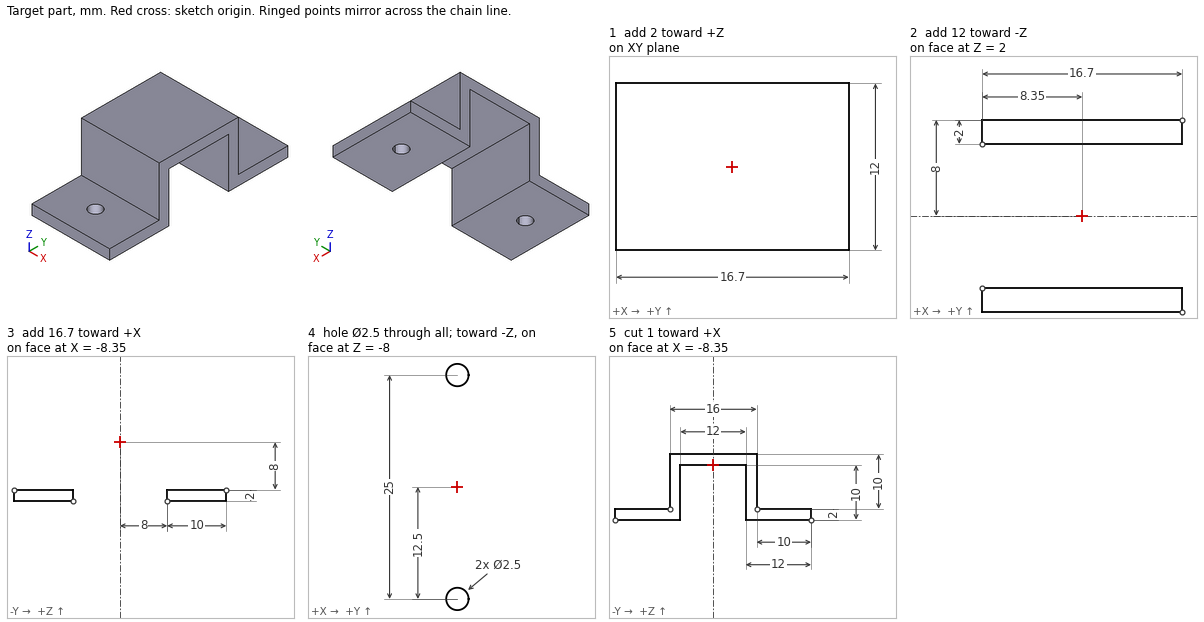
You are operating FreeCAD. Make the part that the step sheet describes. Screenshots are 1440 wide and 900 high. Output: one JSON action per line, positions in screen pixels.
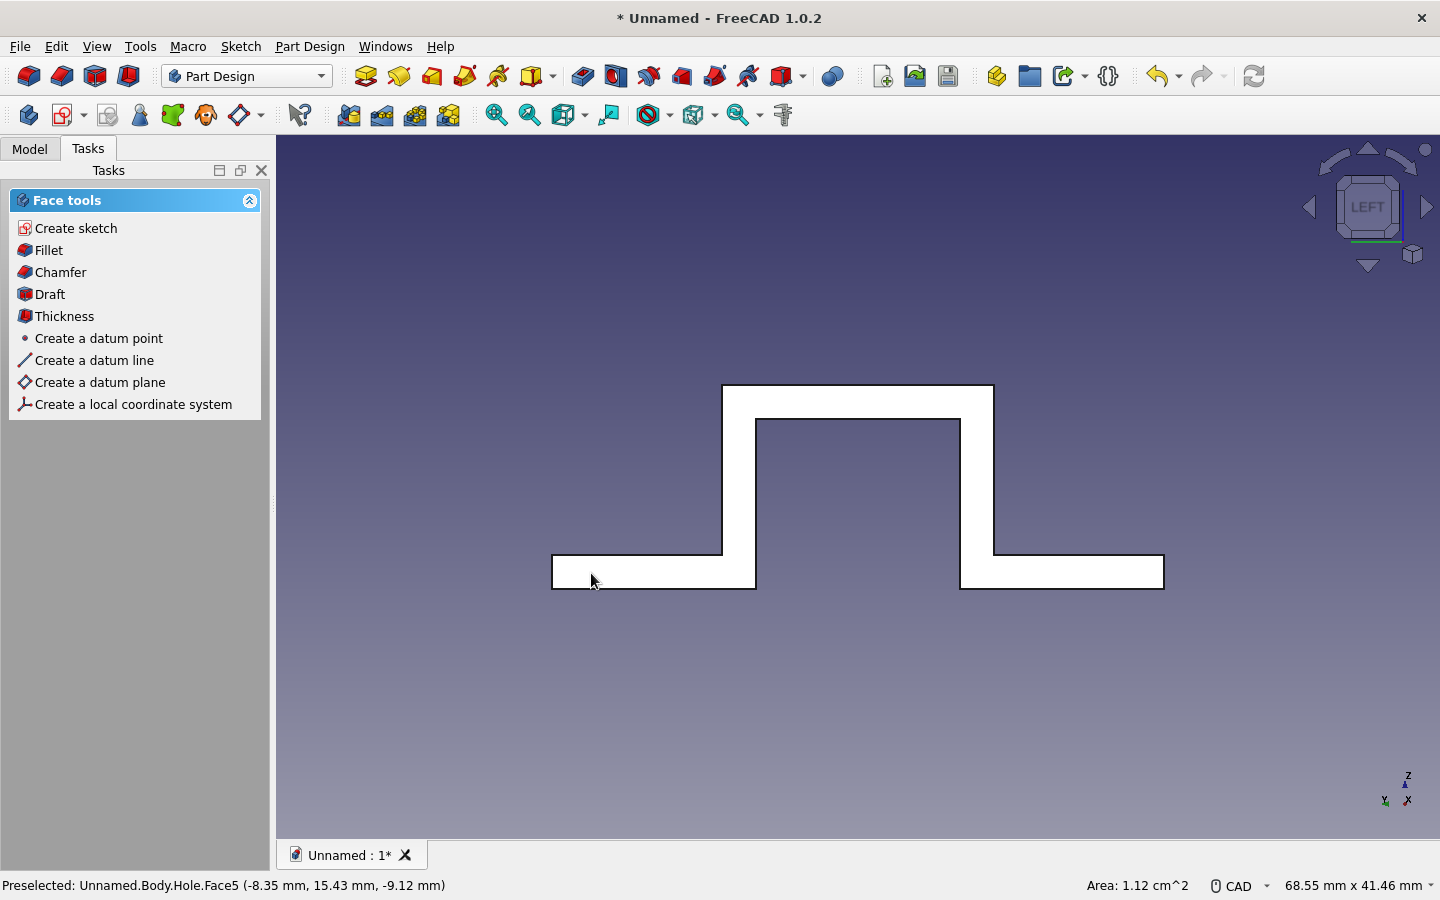
{"action": "left_click", "coordinate": [62, 116]}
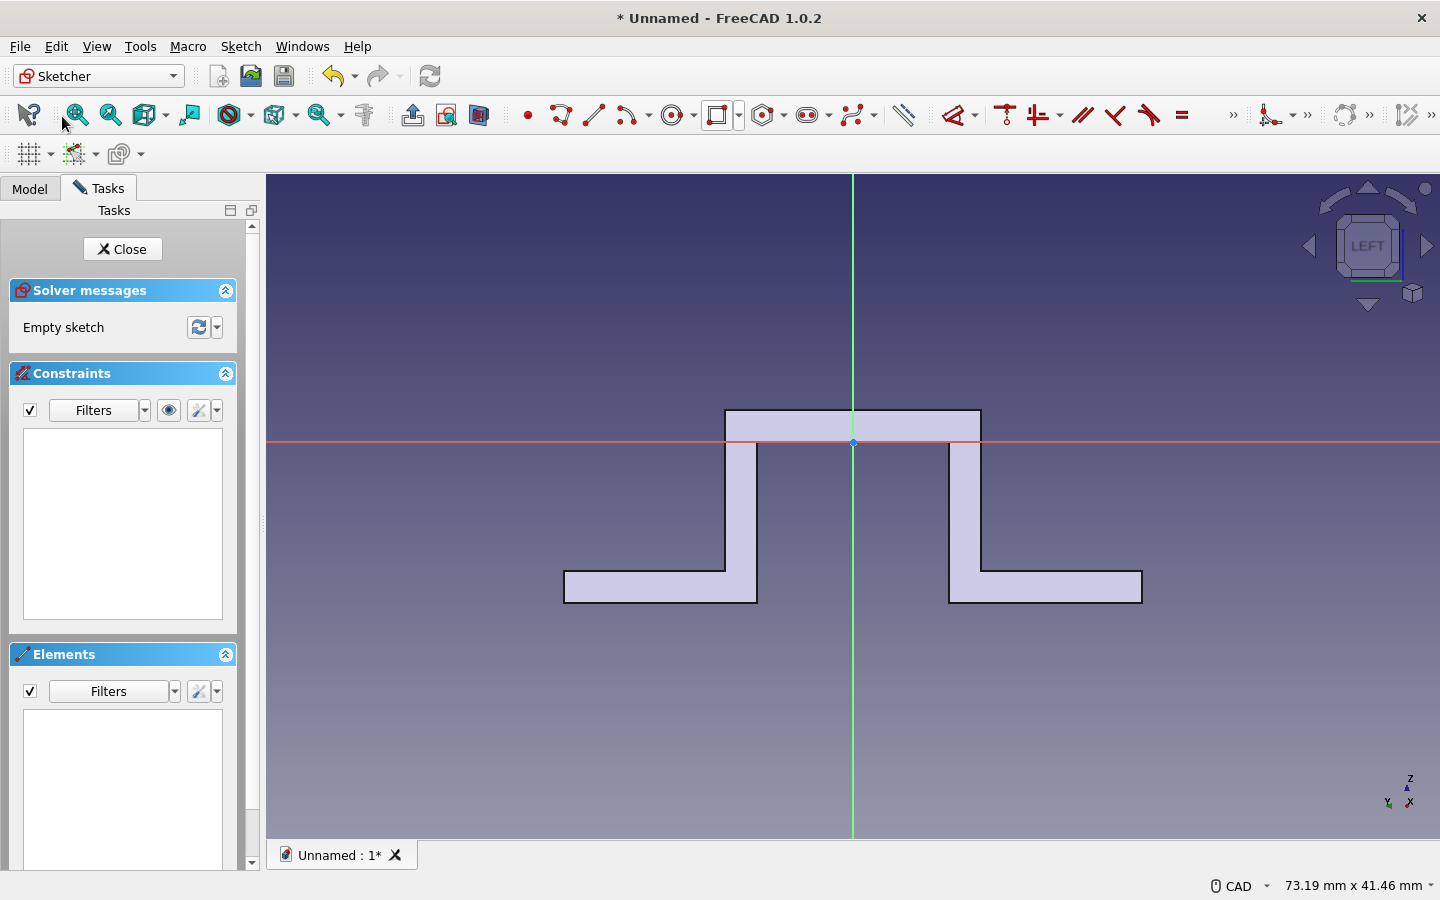
{"action": "left_click", "coordinate": [561, 116]}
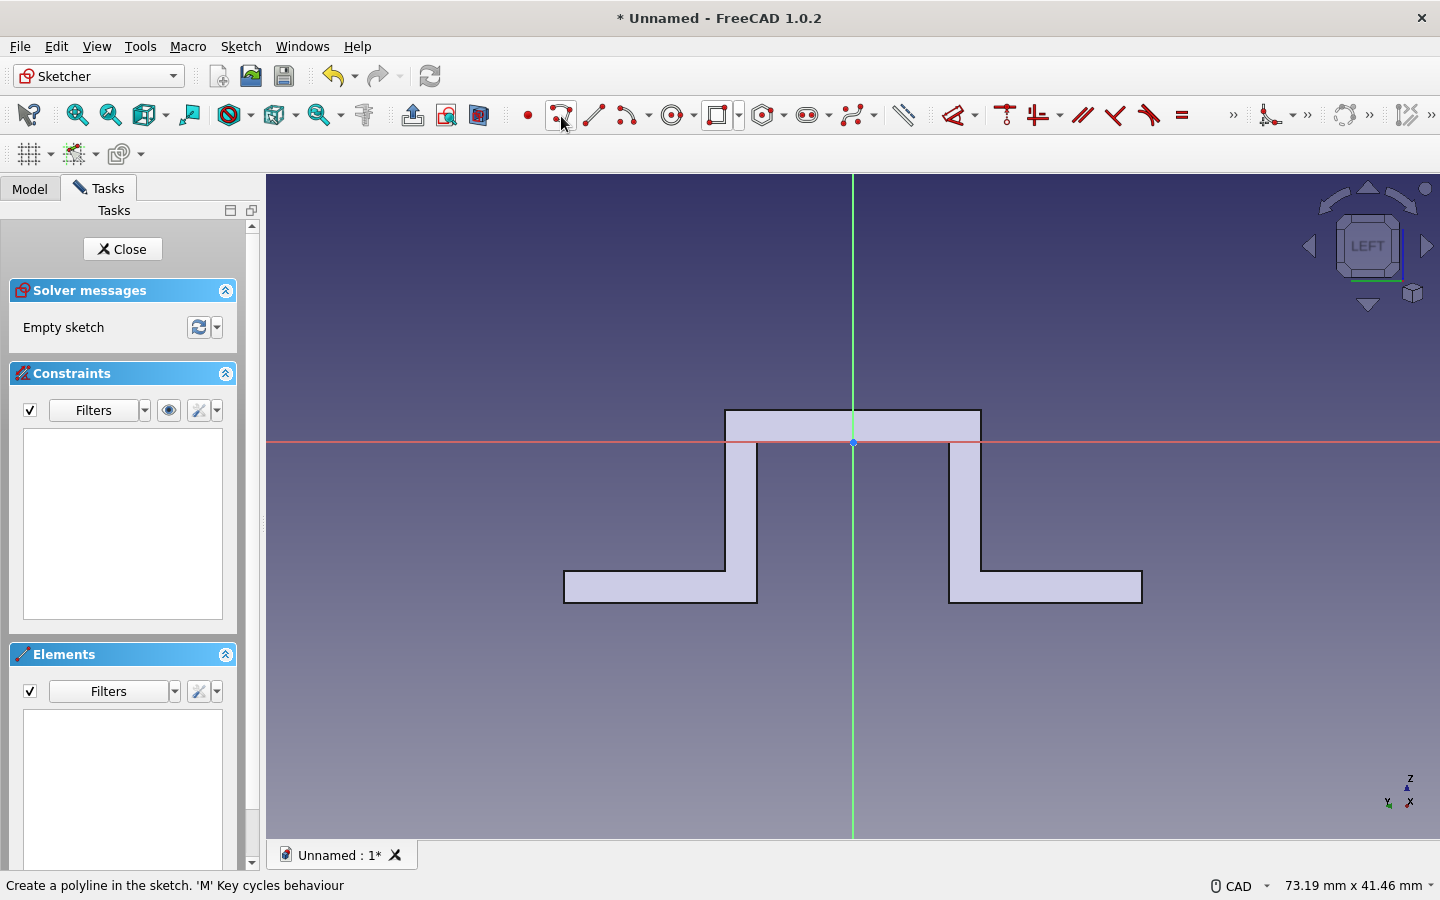
{"action": "left_click", "coordinate": [757, 442]}
{"action": "left_click", "coordinate": [949, 451]}
{"action": "left_click", "coordinate": [949, 603]}
{"action": "left_click", "coordinate": [1142, 603]}
{"action": "left_click", "coordinate": [1142, 571]}
{"action": "left_click", "coordinate": [981, 571]}
{"action": "left_click", "coordinate": [981, 410]}
{"action": "left_click", "coordinate": [725, 410]}
{"action": "left_click", "coordinate": [725, 571]}
{"action": "left_click", "coordinate": [564, 571]}
{"action": "left_click", "coordinate": [564, 603]}
{"action": "left_click", "coordinate": [757, 603]}
{"action": "left_click", "coordinate": [757, 442]}
{"action": "key", "text": "Escape"}
{"action": "key", "text": "Escape"}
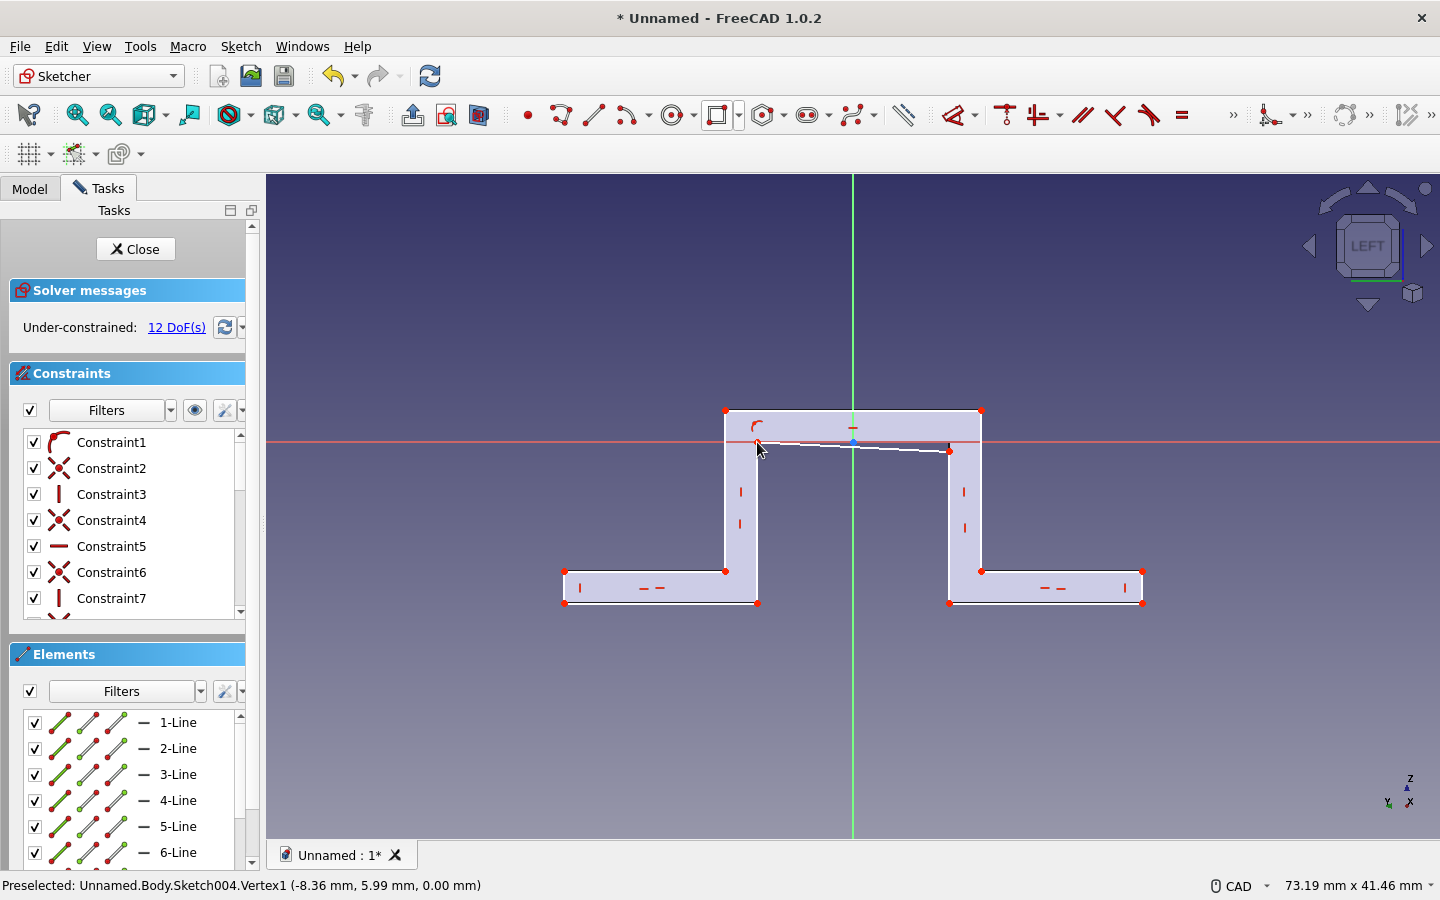
{"action": "left_click", "coordinate": [815, 445]}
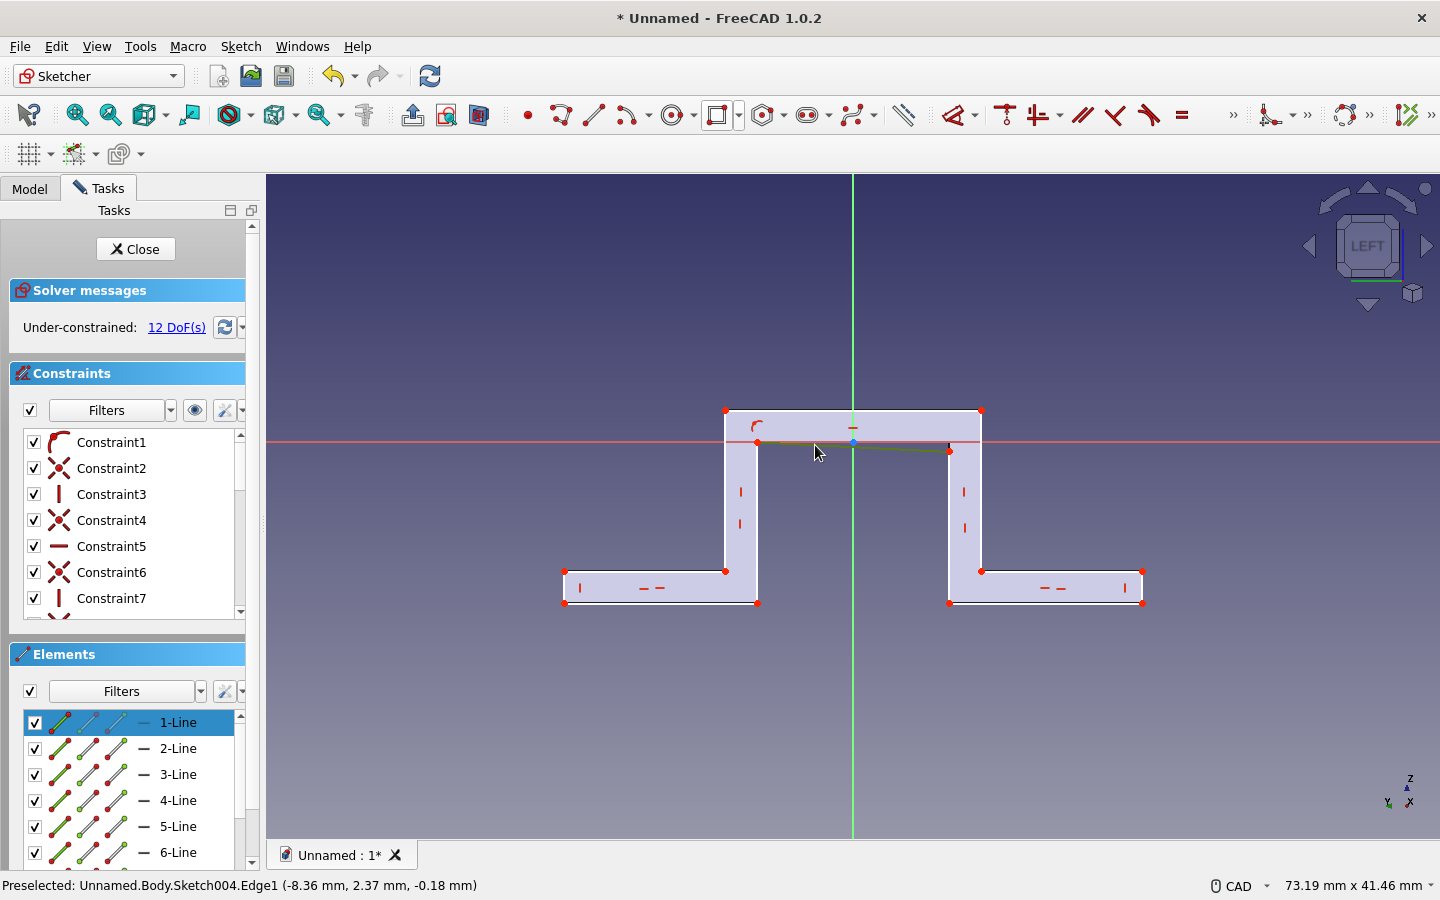
{"action": "key", "text": "h"}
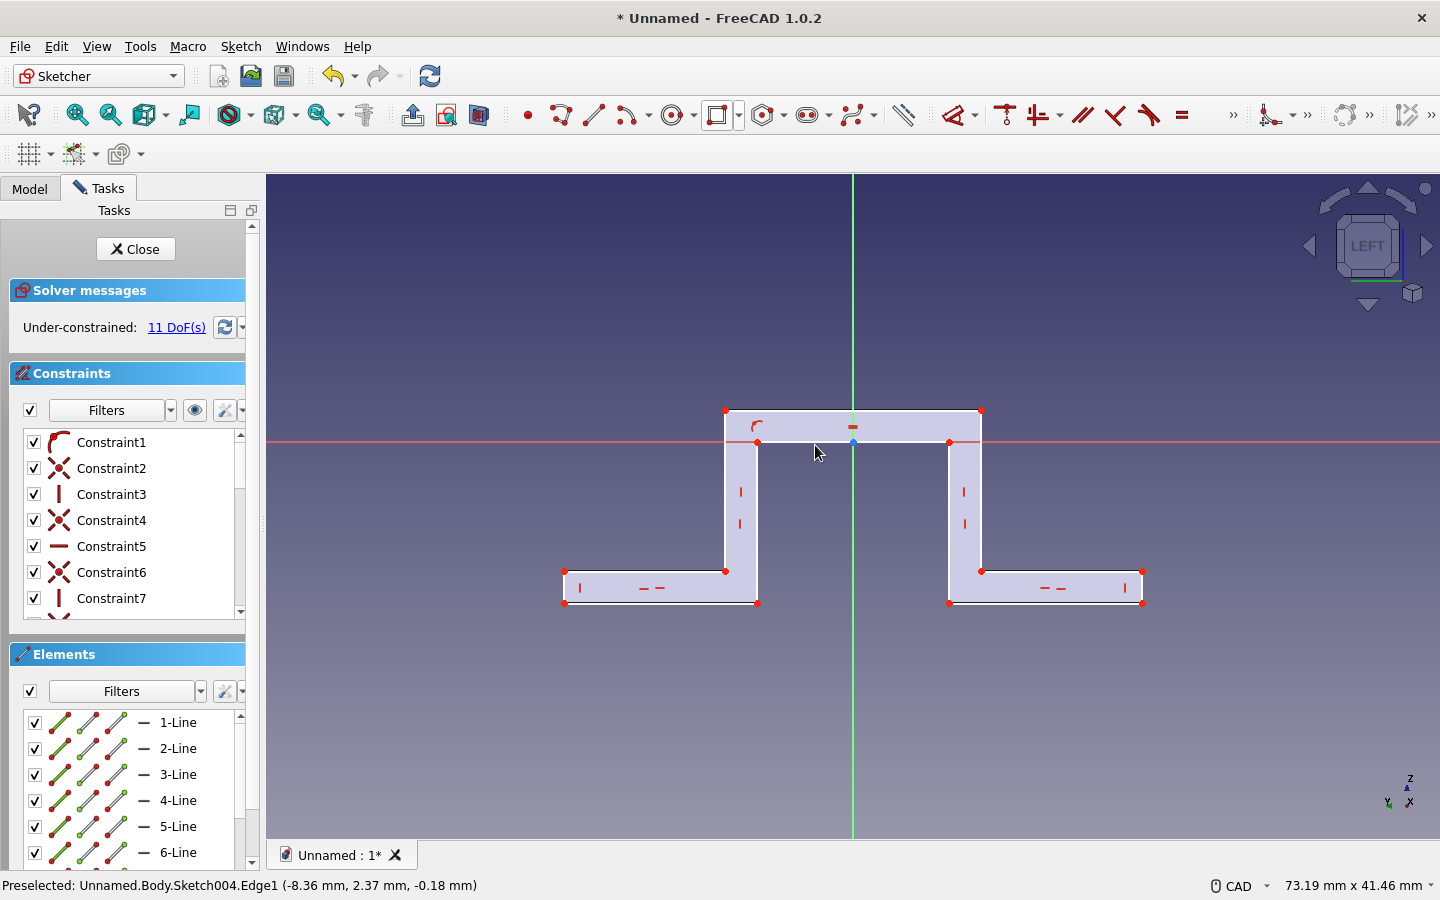
{"action": "left_click", "coordinate": [981, 572]}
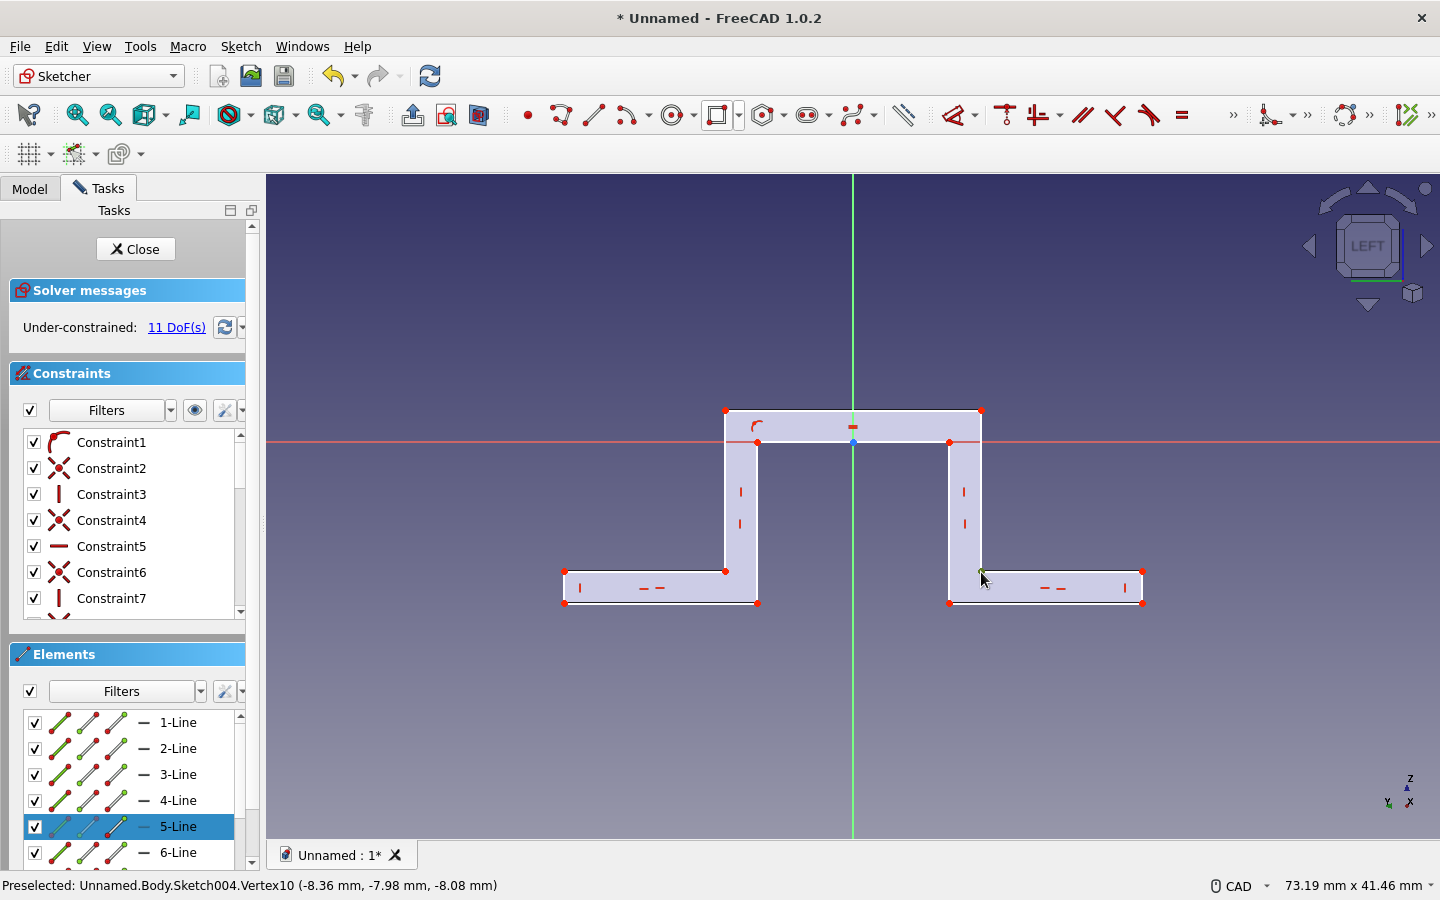
{"action": "left_click", "coordinate": [725, 572]}